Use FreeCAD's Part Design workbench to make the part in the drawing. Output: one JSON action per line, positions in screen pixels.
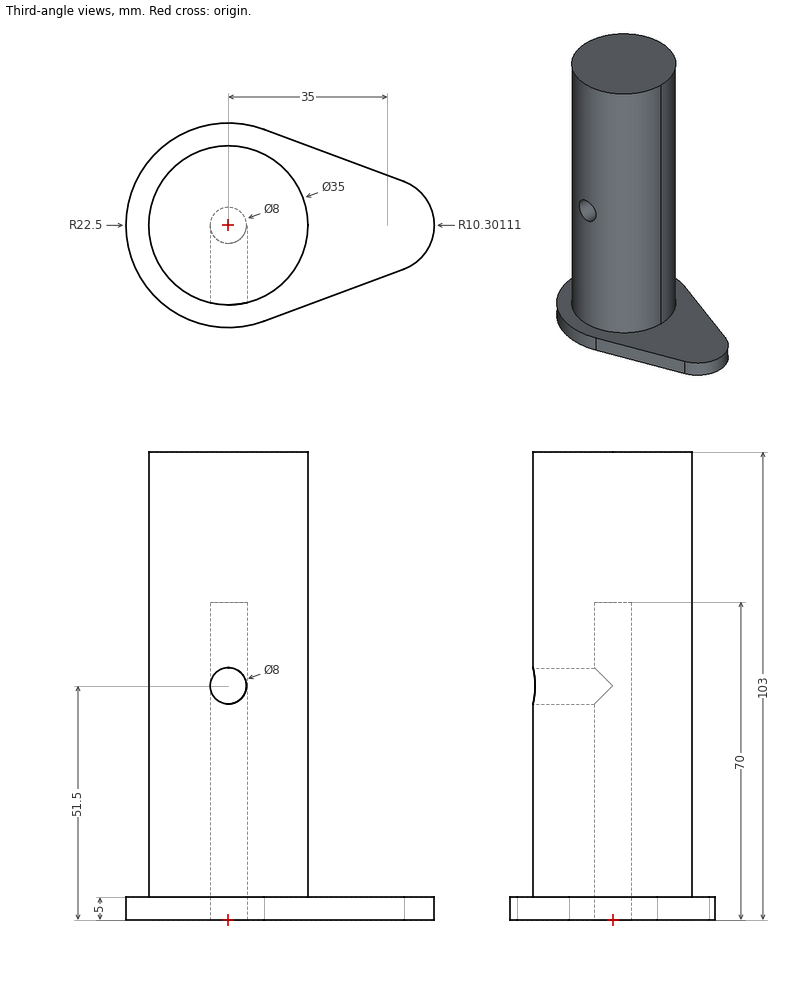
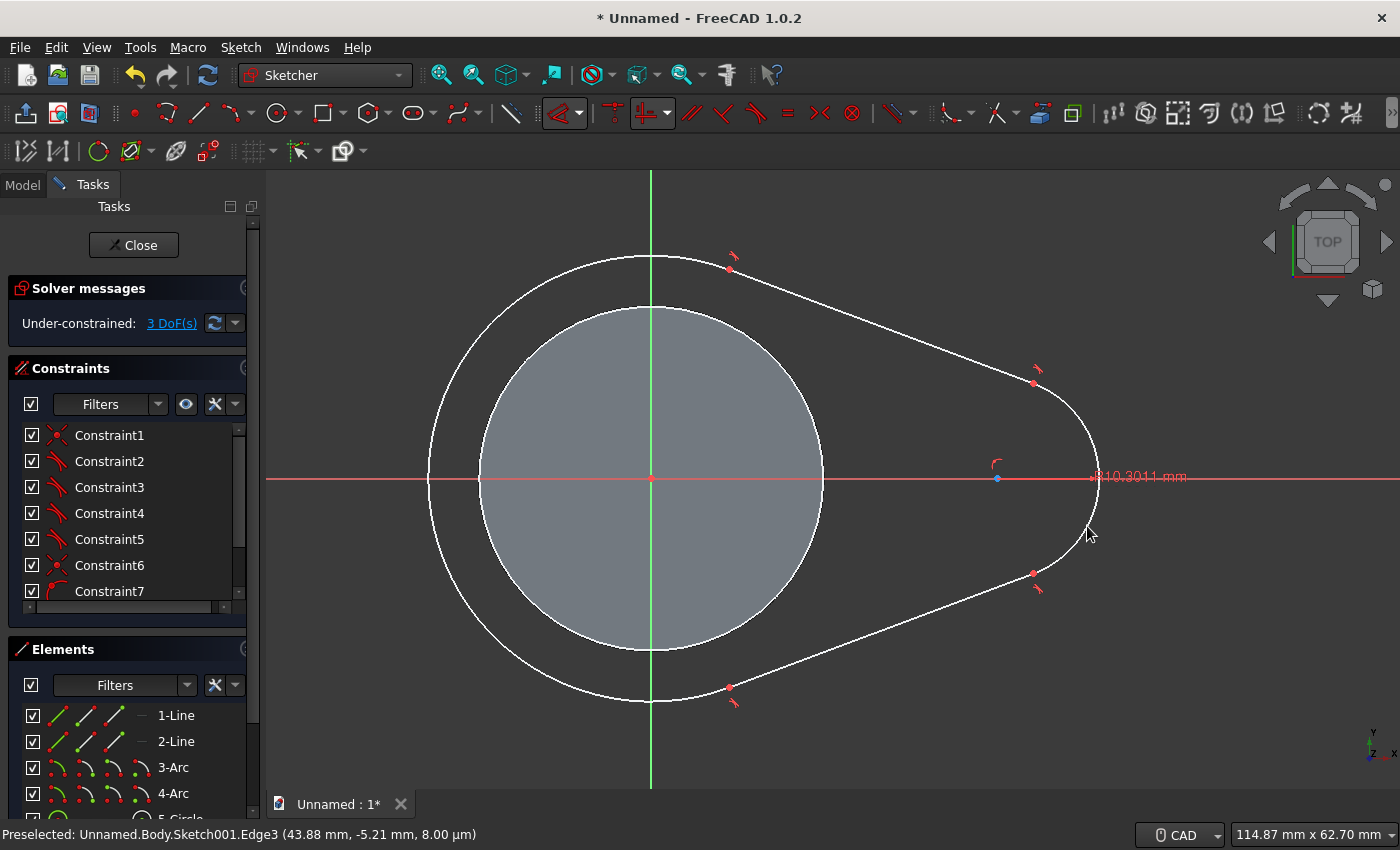
{"action": "left_click", "coordinate": [491, 323]}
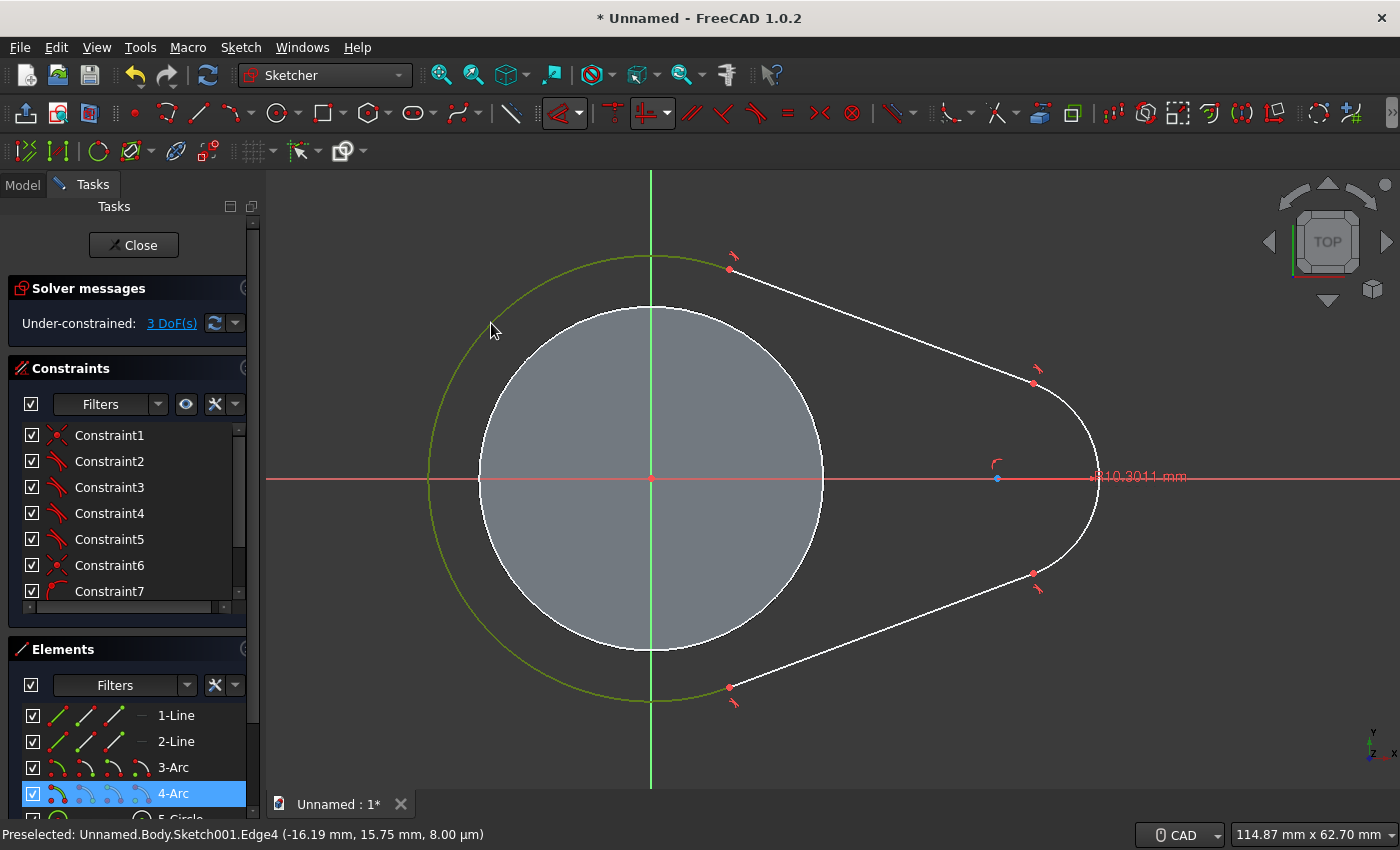
{"action": "left_click", "coordinate": [582, 114]}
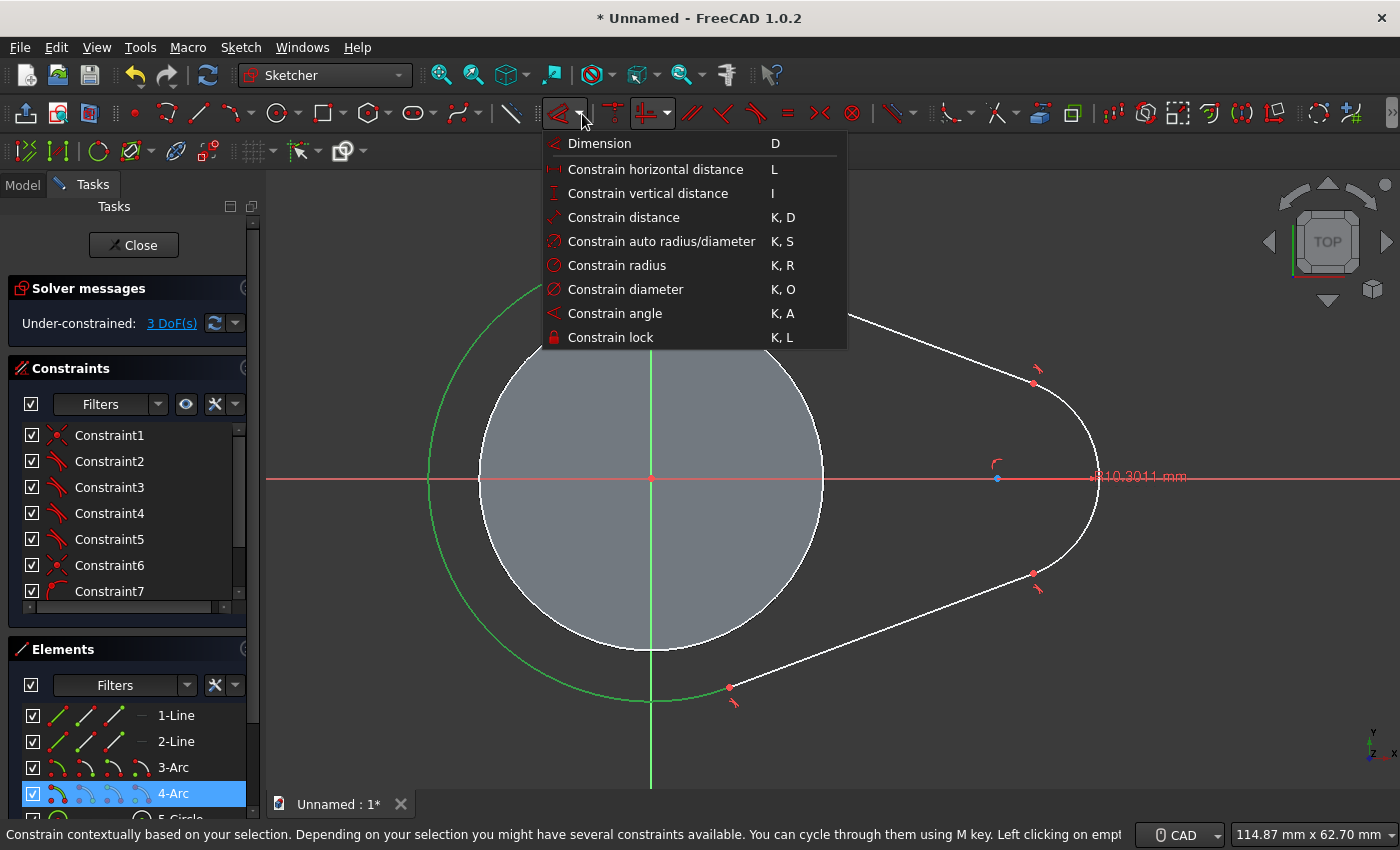
{"action": "left_click", "coordinate": [695, 265]}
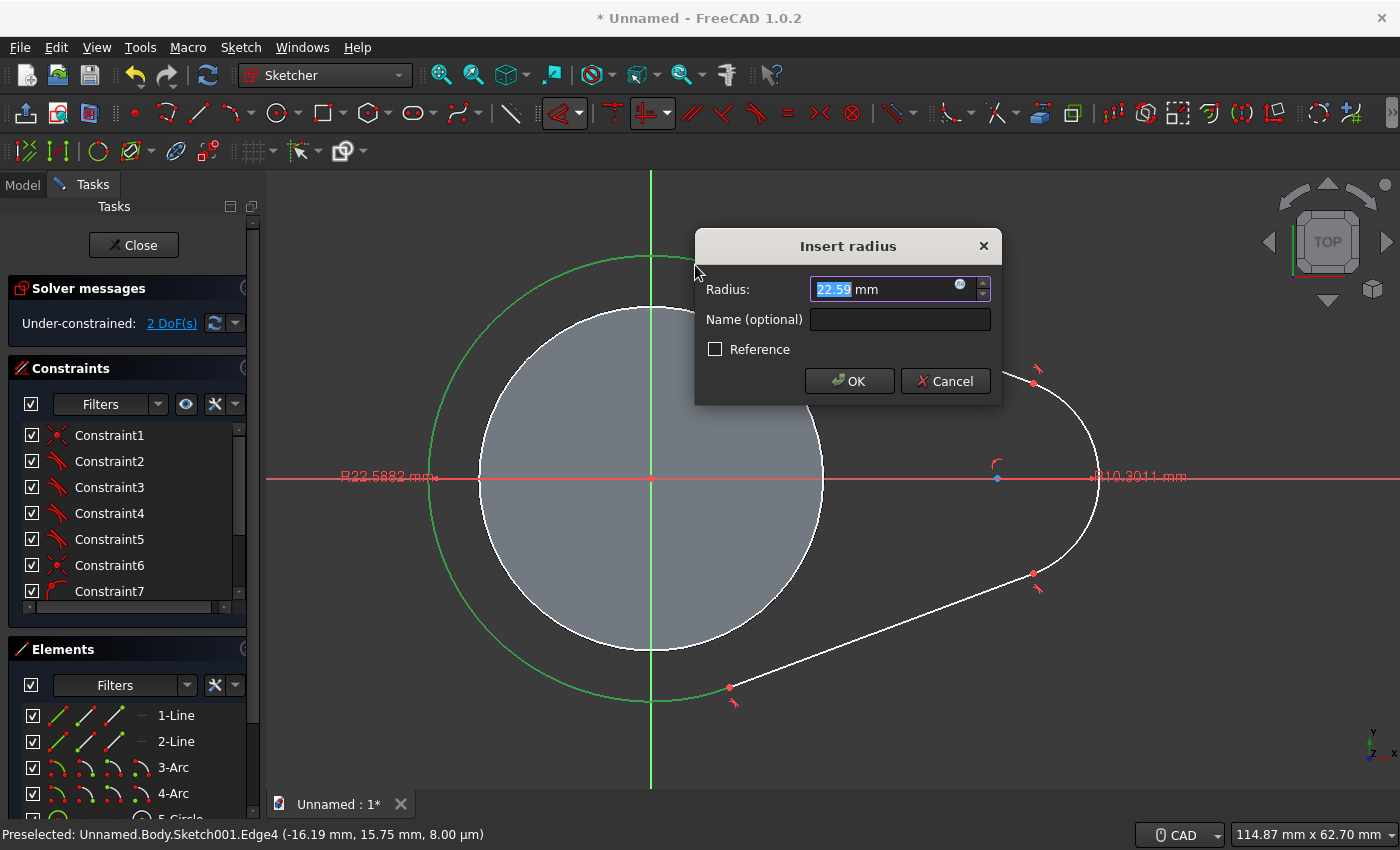
{"action": "type", "text": "22.5"}
{"action": "key", "text": "Return"}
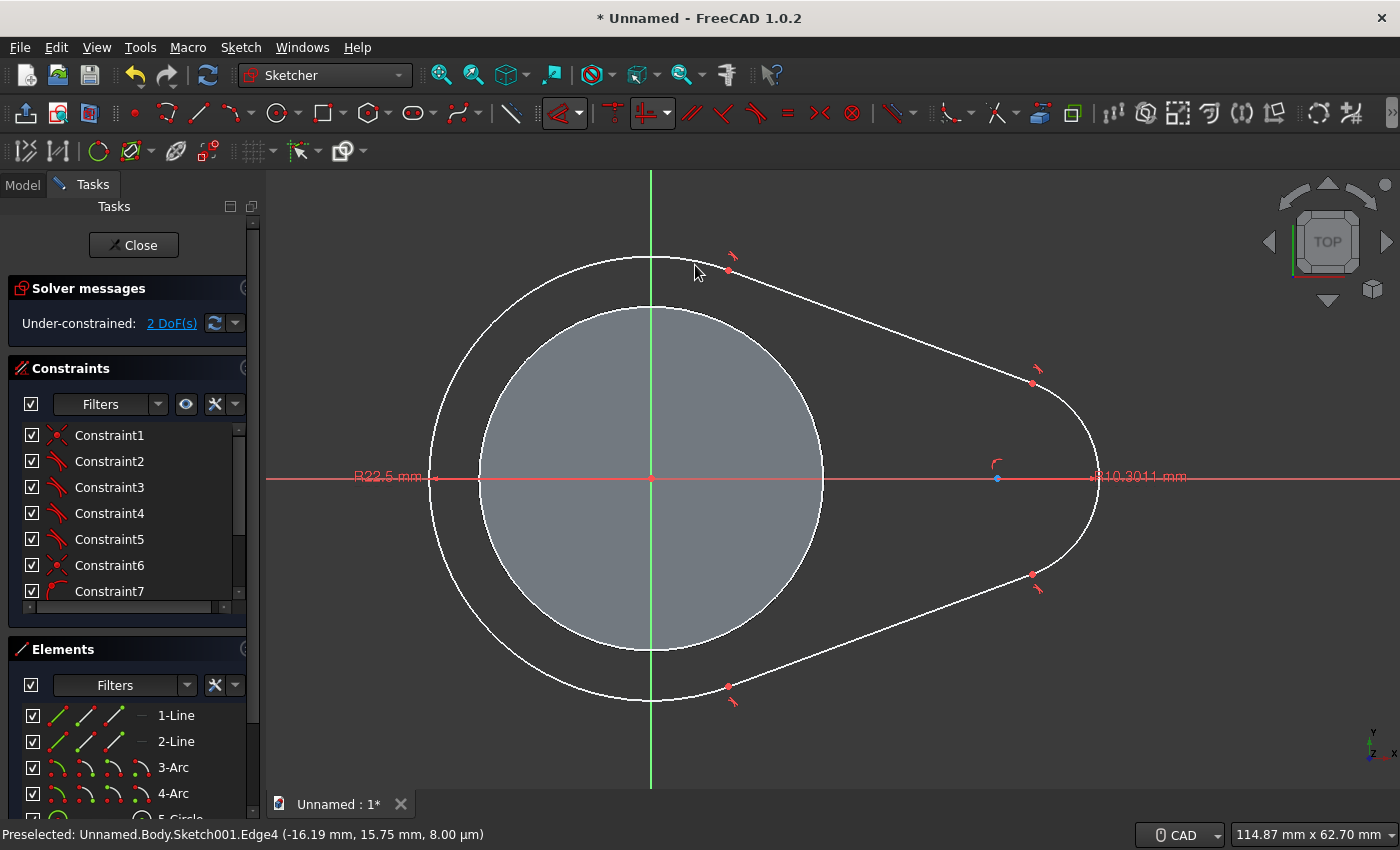
{"action": "left_click", "coordinate": [773, 357]}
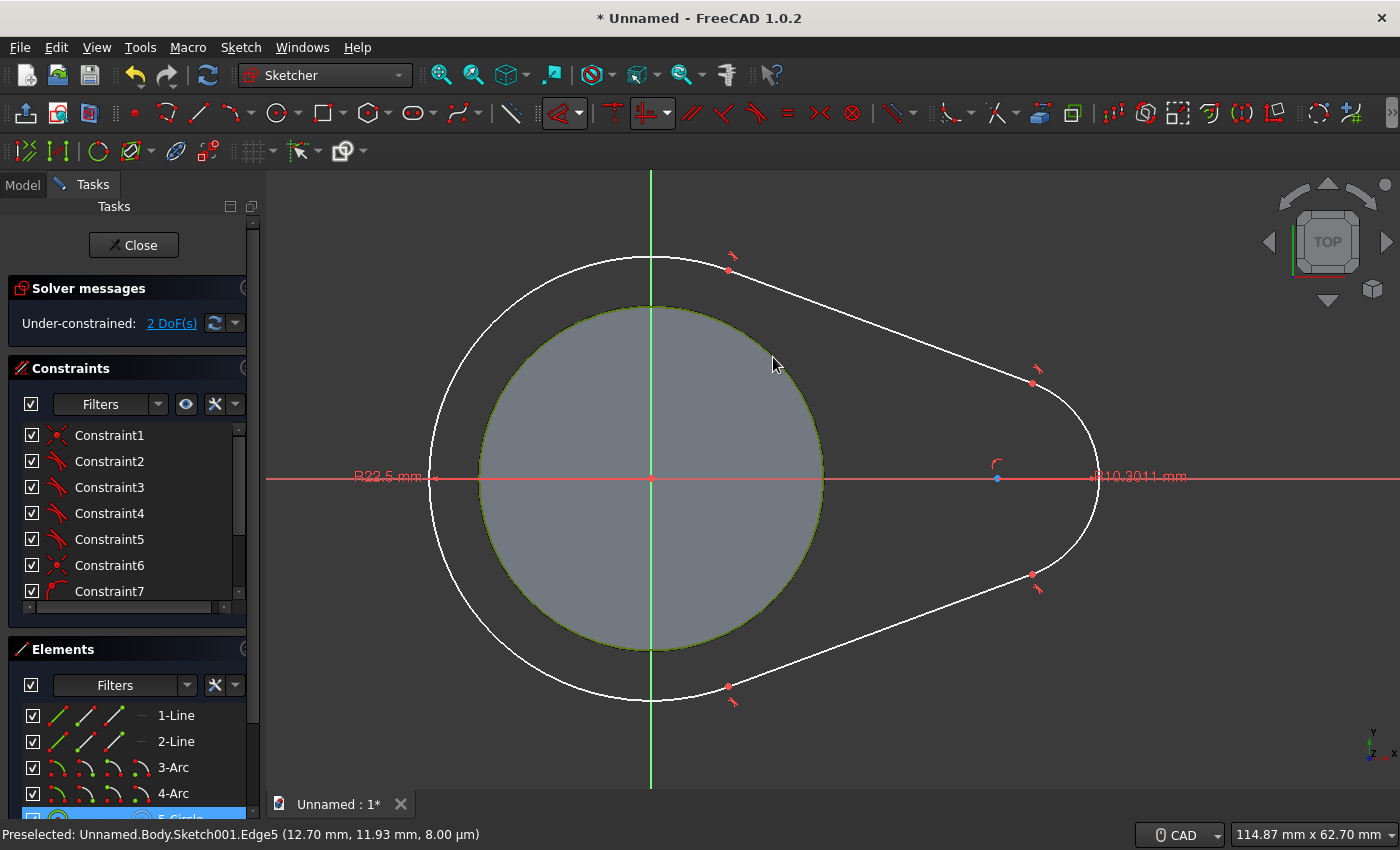
{"action": "left_click", "coordinate": [582, 114]}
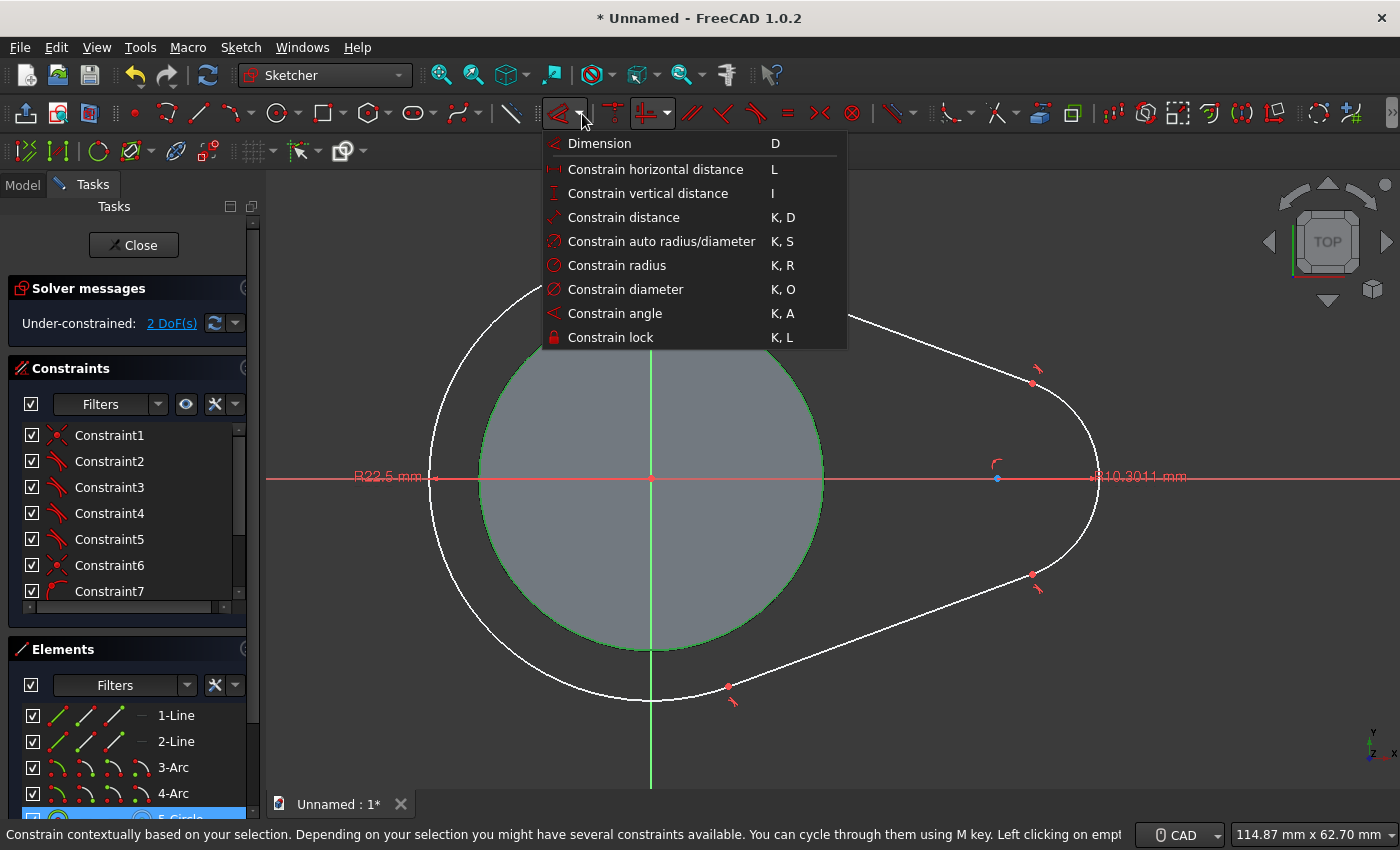
{"action": "left_click", "coordinate": [695, 289]}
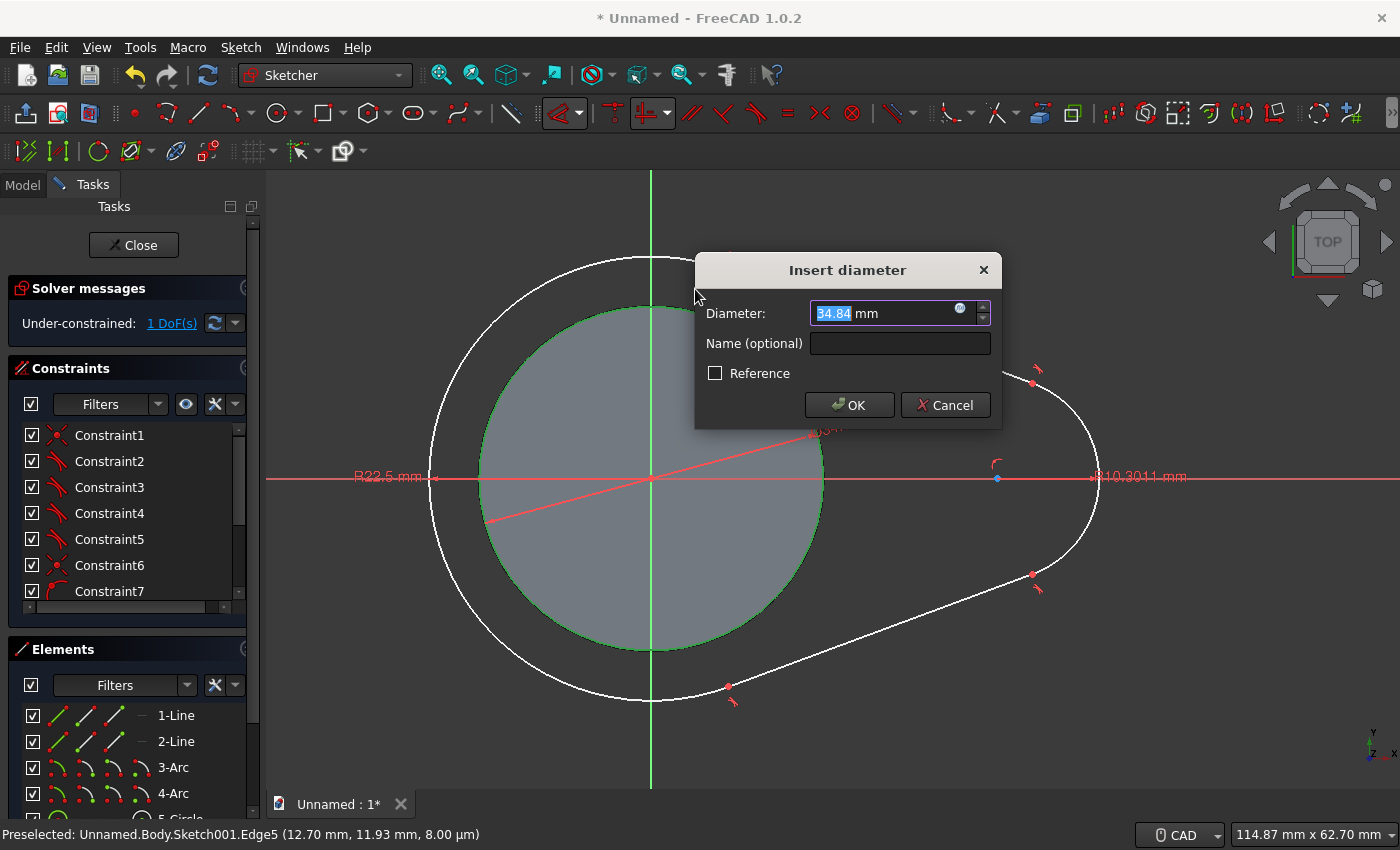
{"action": "type", "text": "35"}
{"action": "key", "text": "Return"}